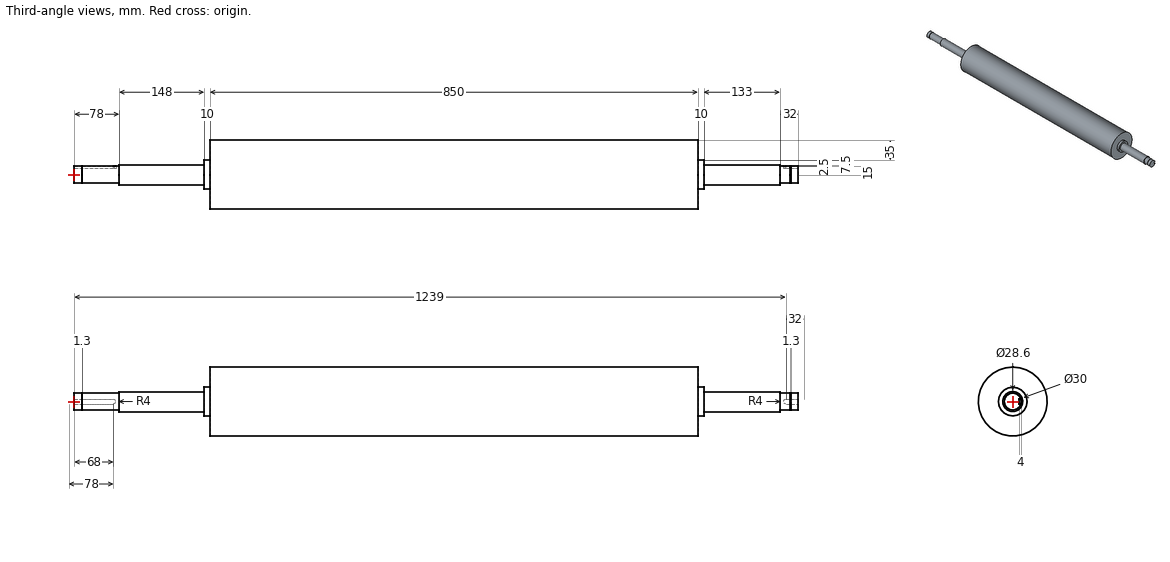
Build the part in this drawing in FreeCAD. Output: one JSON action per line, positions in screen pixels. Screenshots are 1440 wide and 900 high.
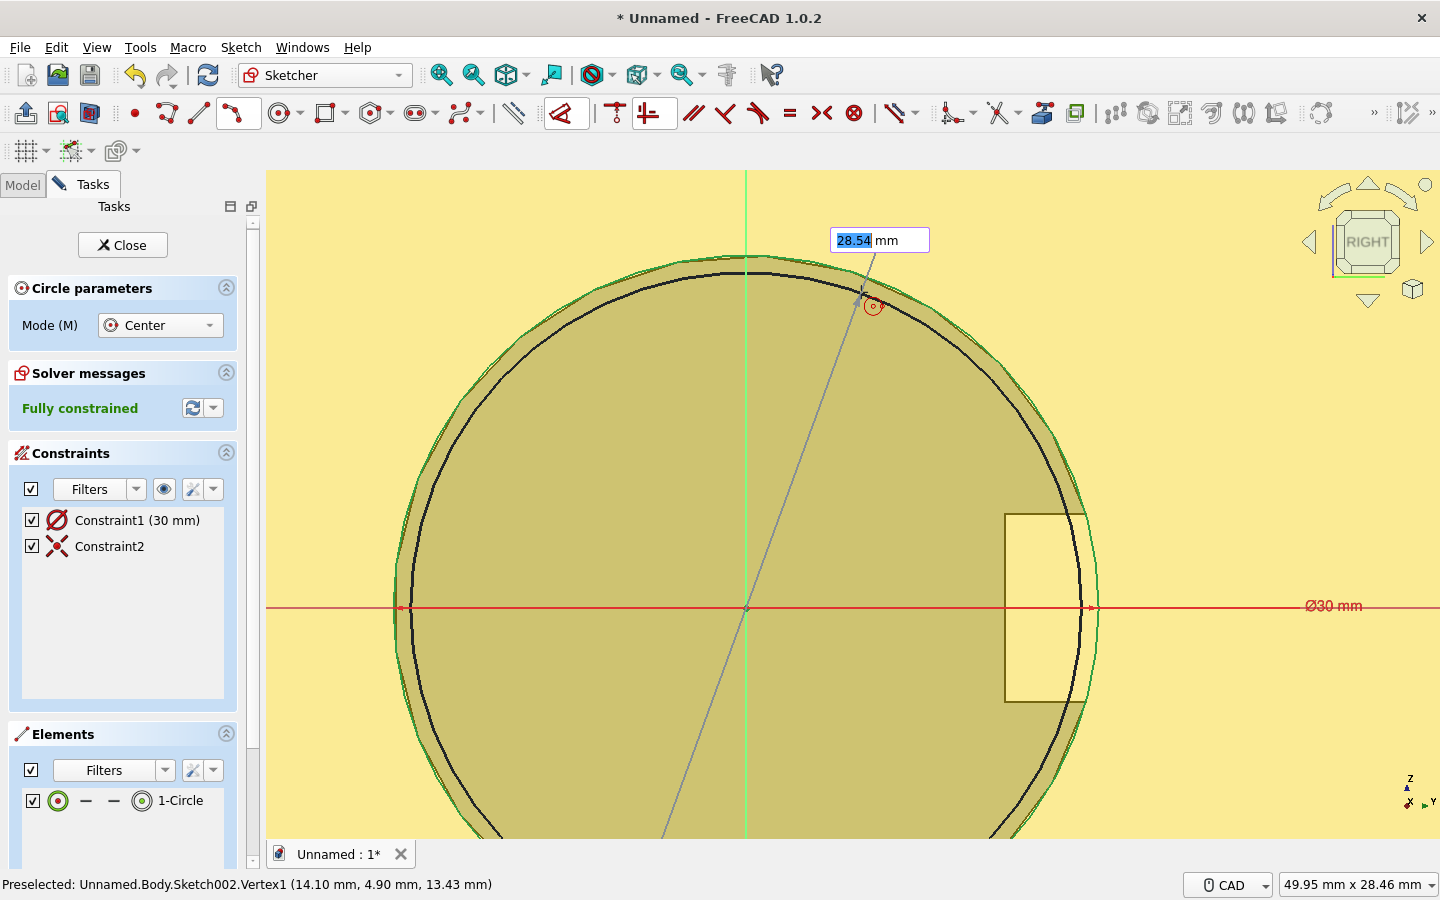
{"action": "type", "text": "28.6"}
{"action": "key", "text": "Return"}
{"action": "key", "text": "Escape"}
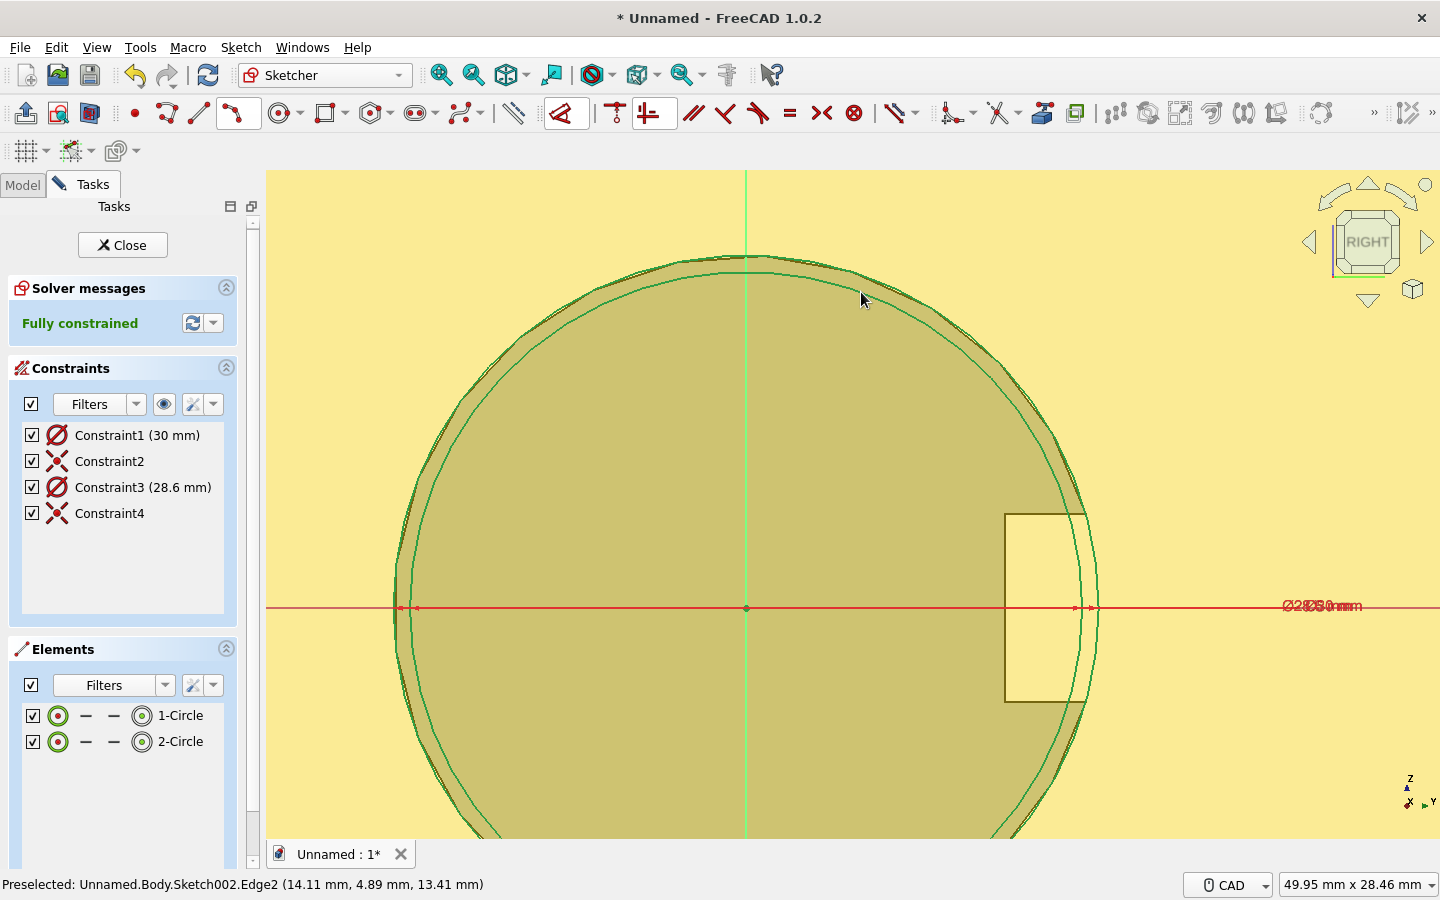
{"action": "left_click", "coordinate": [123, 245]}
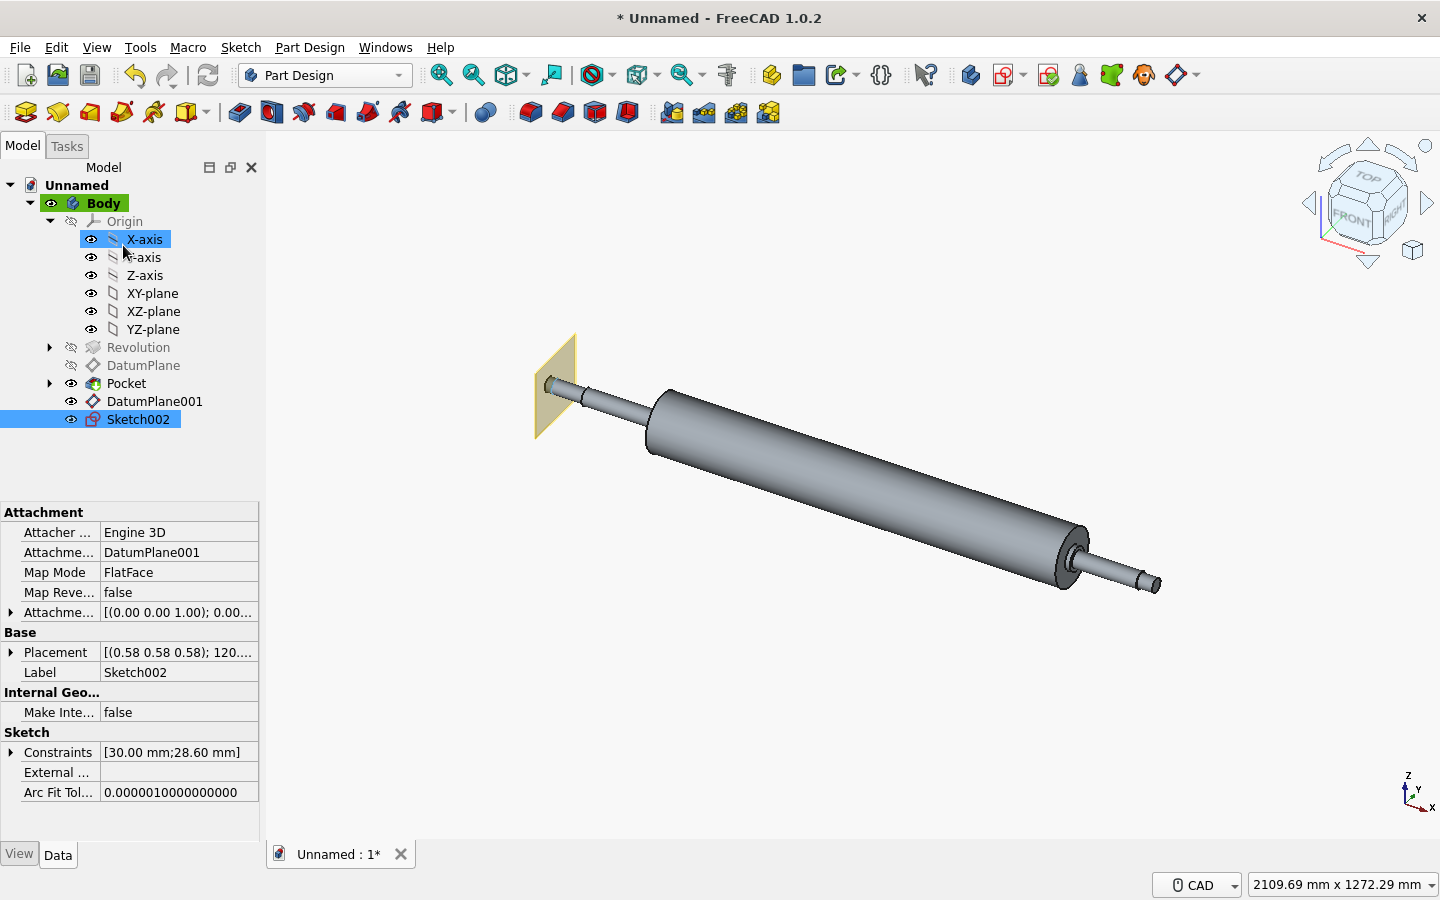
{"action": "left_click", "coordinate": [240, 112]}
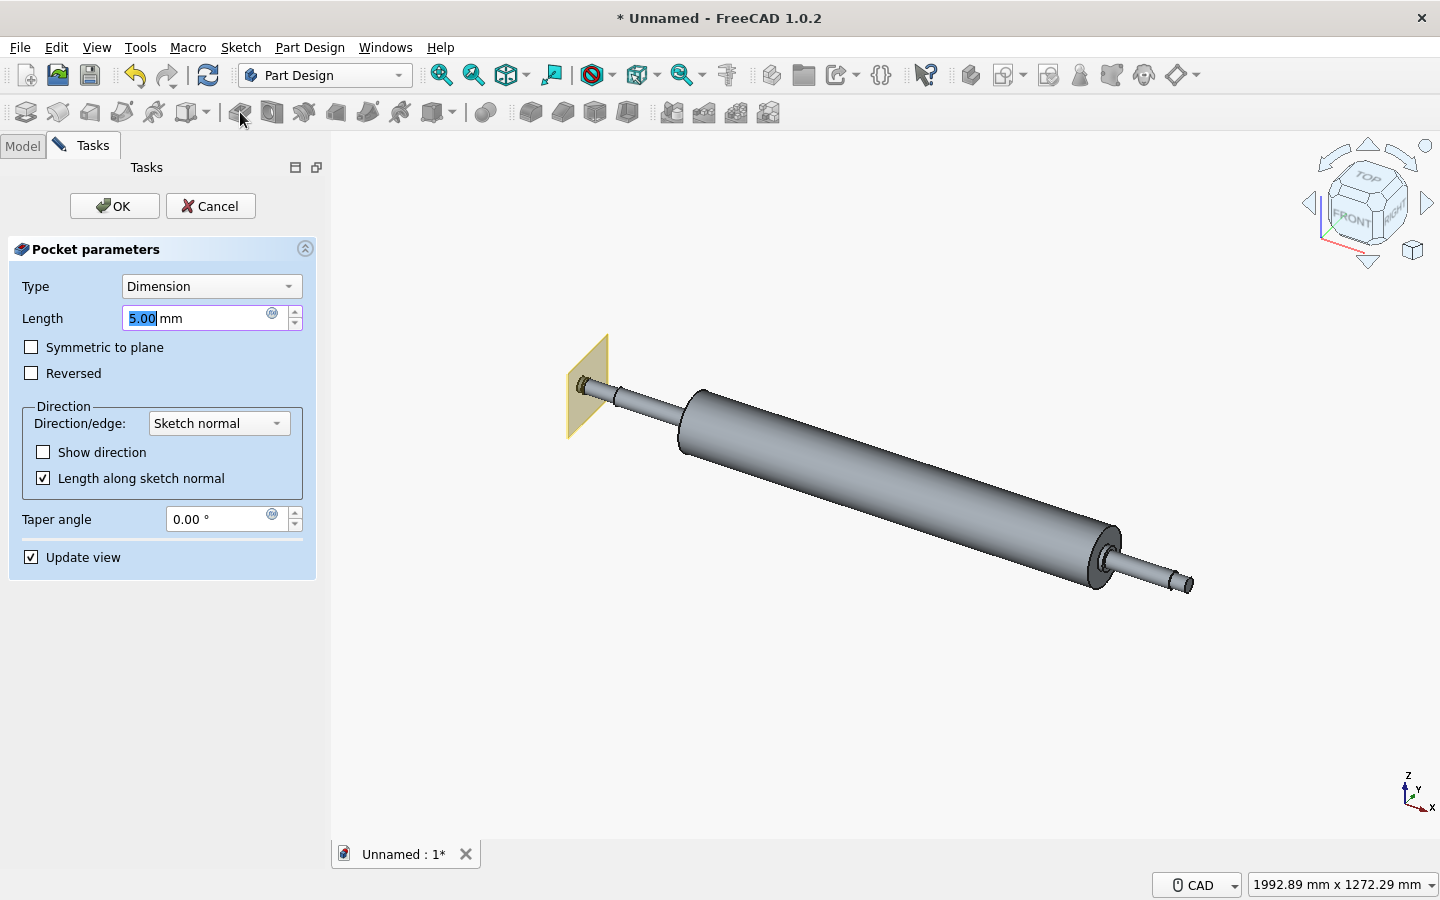
{"action": "type", "text": "1.3"}
{"action": "key", "text": "Tab"}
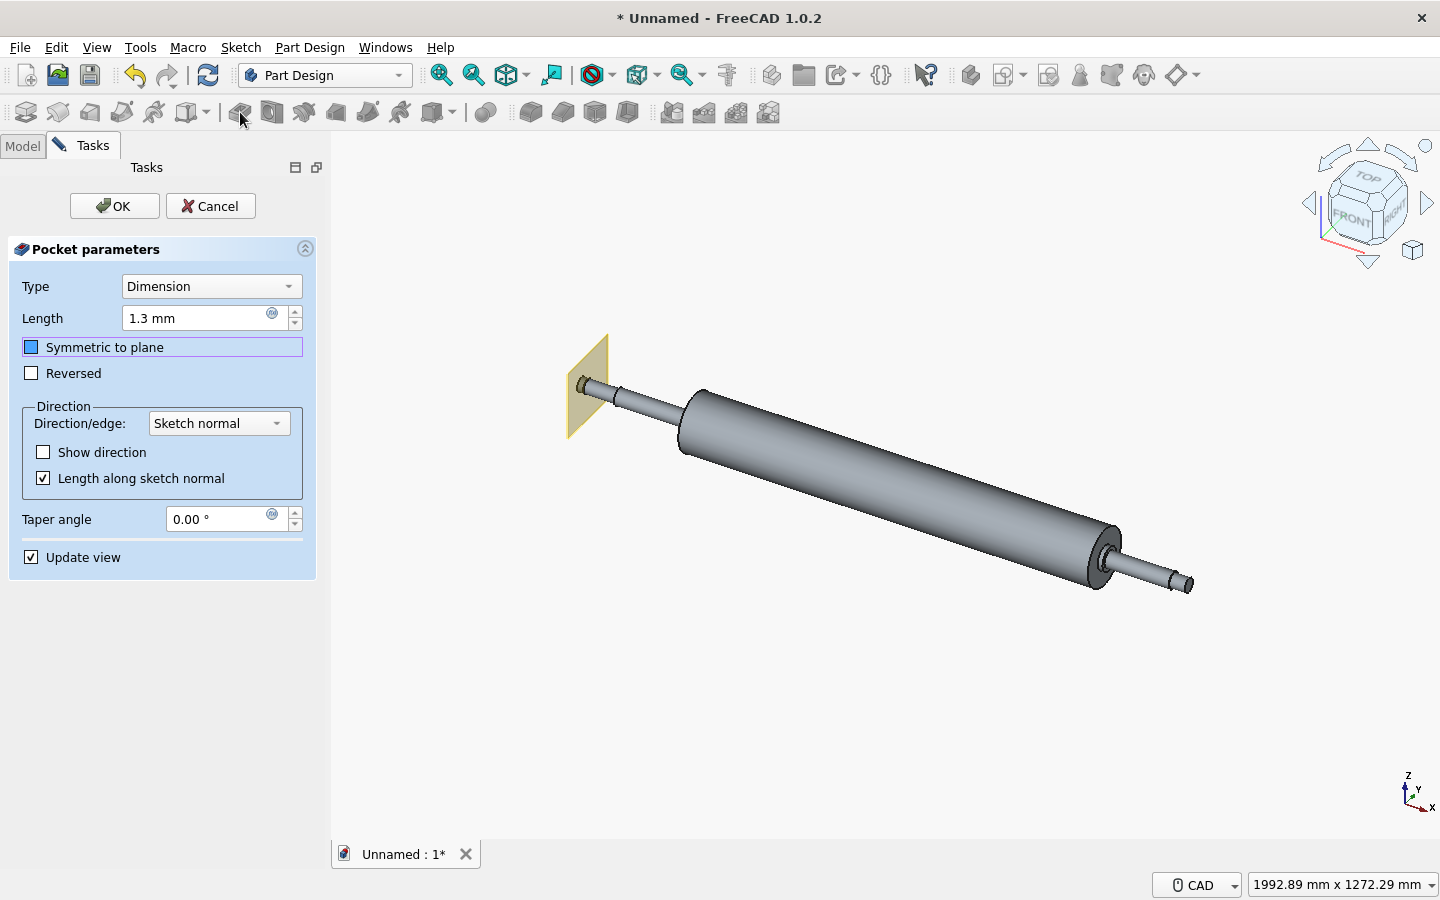
{"action": "left_click", "coordinate": [115, 206]}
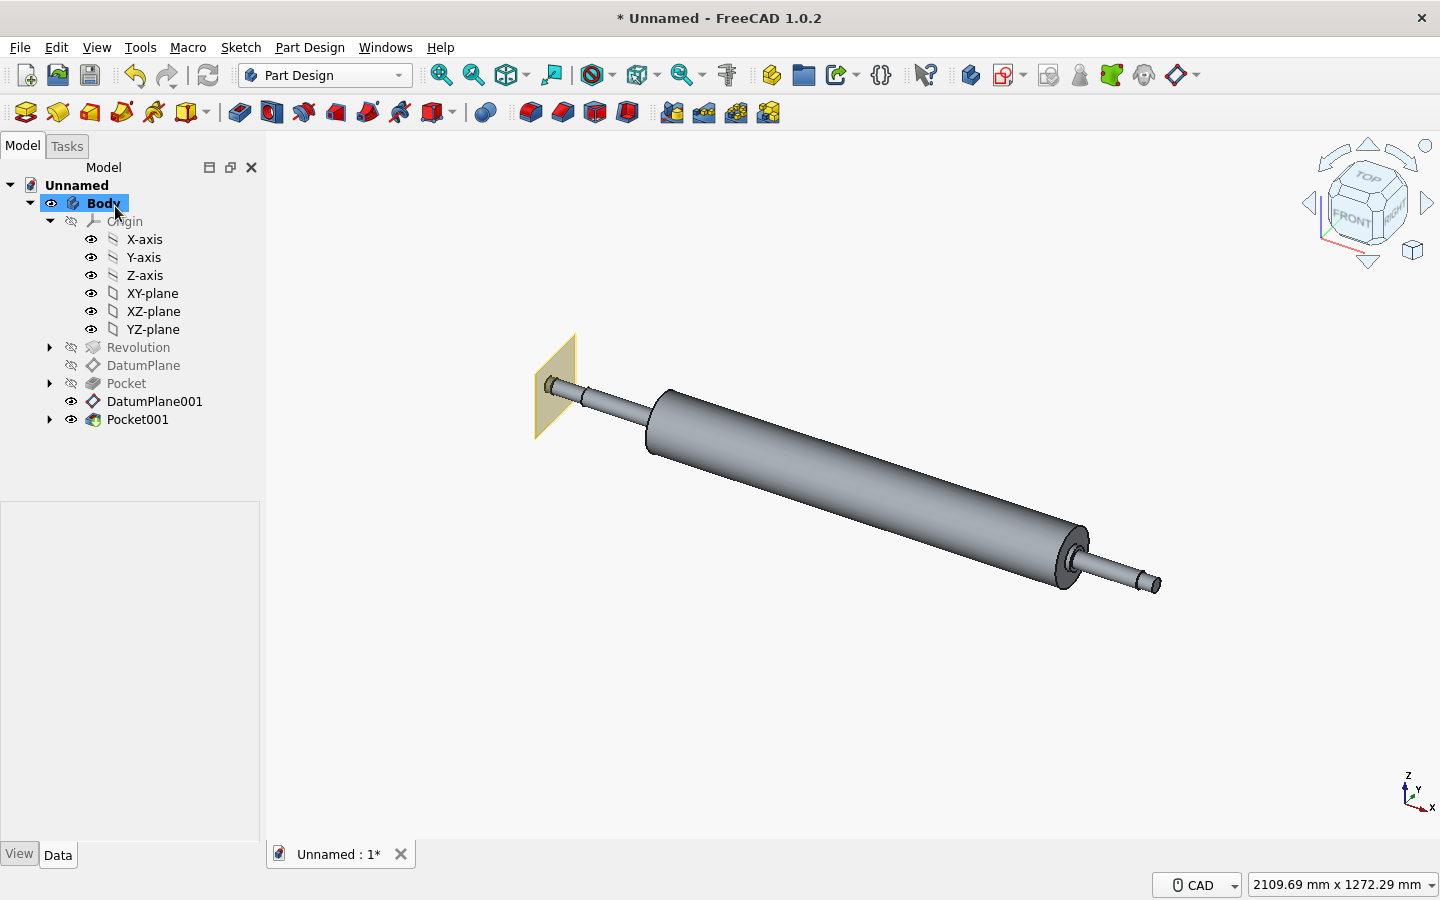
{"action": "left_click", "coordinate": [116, 401]}
{"action": "key", "text": "space"}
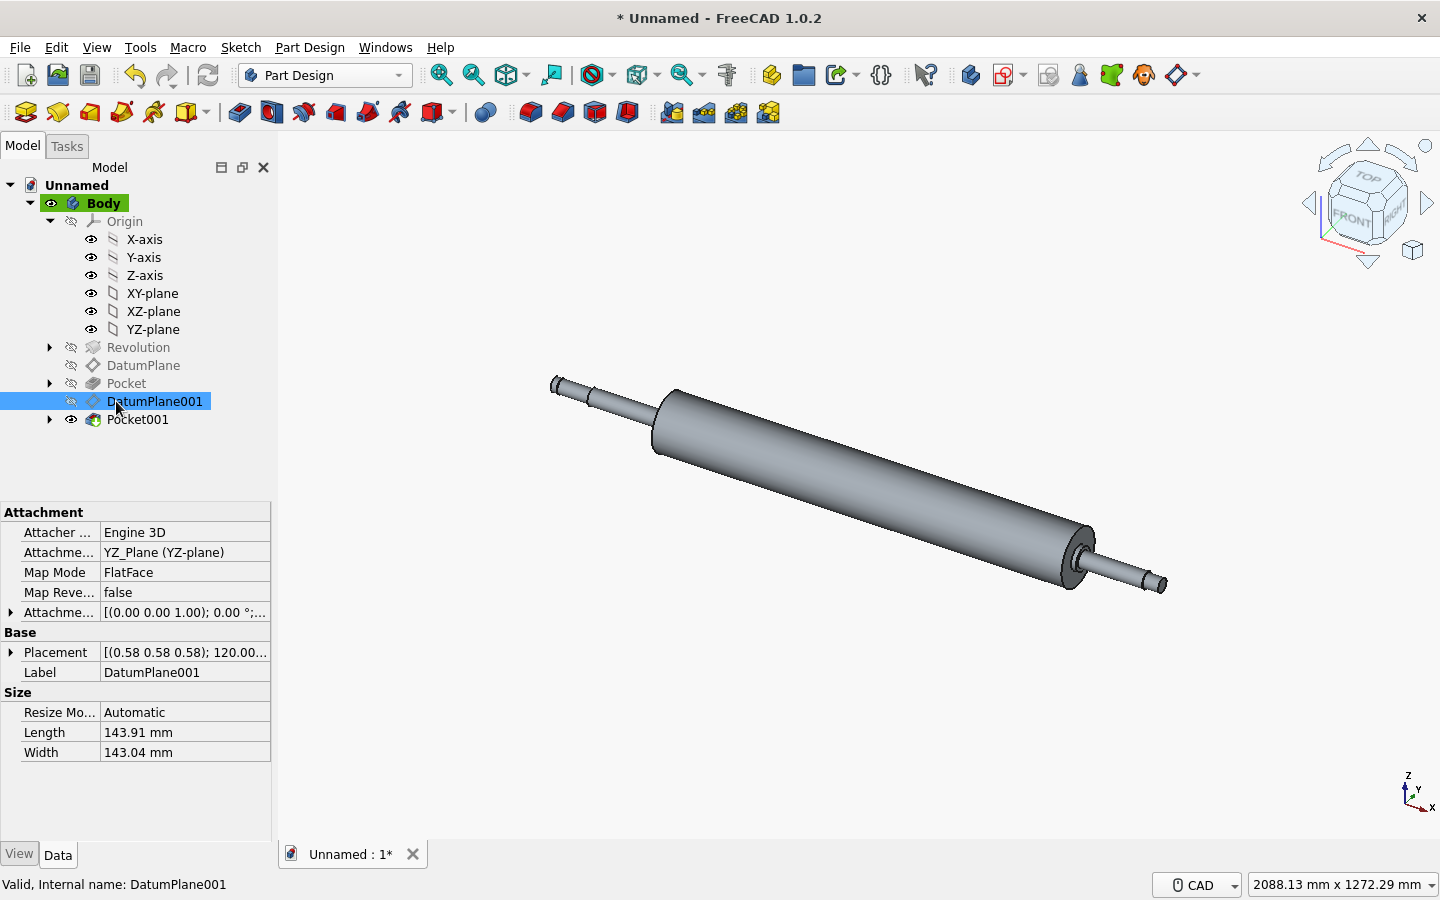
{"action": "left_click", "coordinate": [136, 311]}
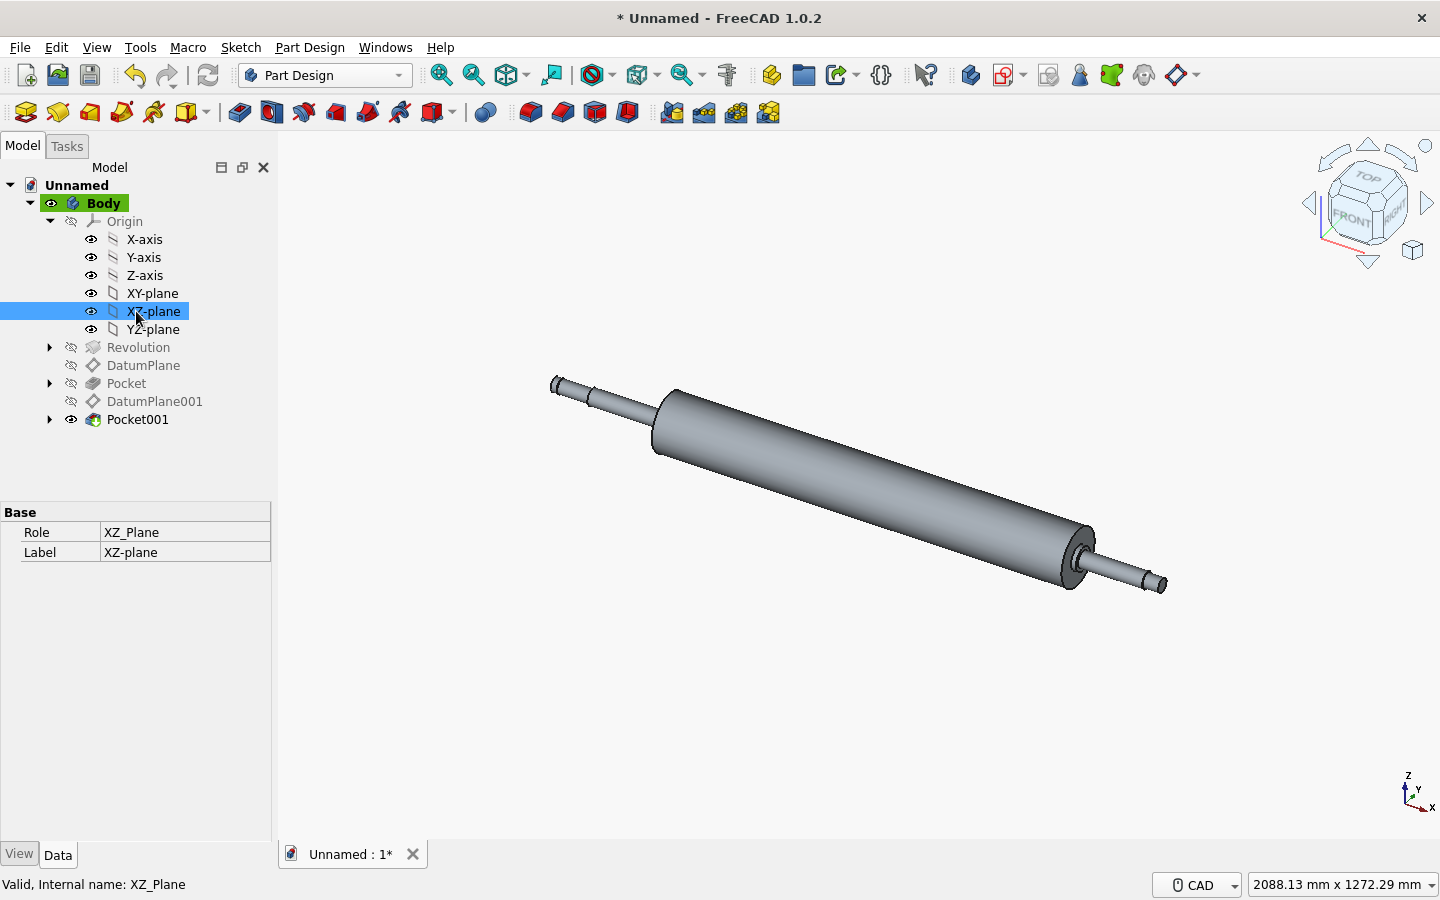
{"action": "left_click", "coordinate": [1176, 76]}